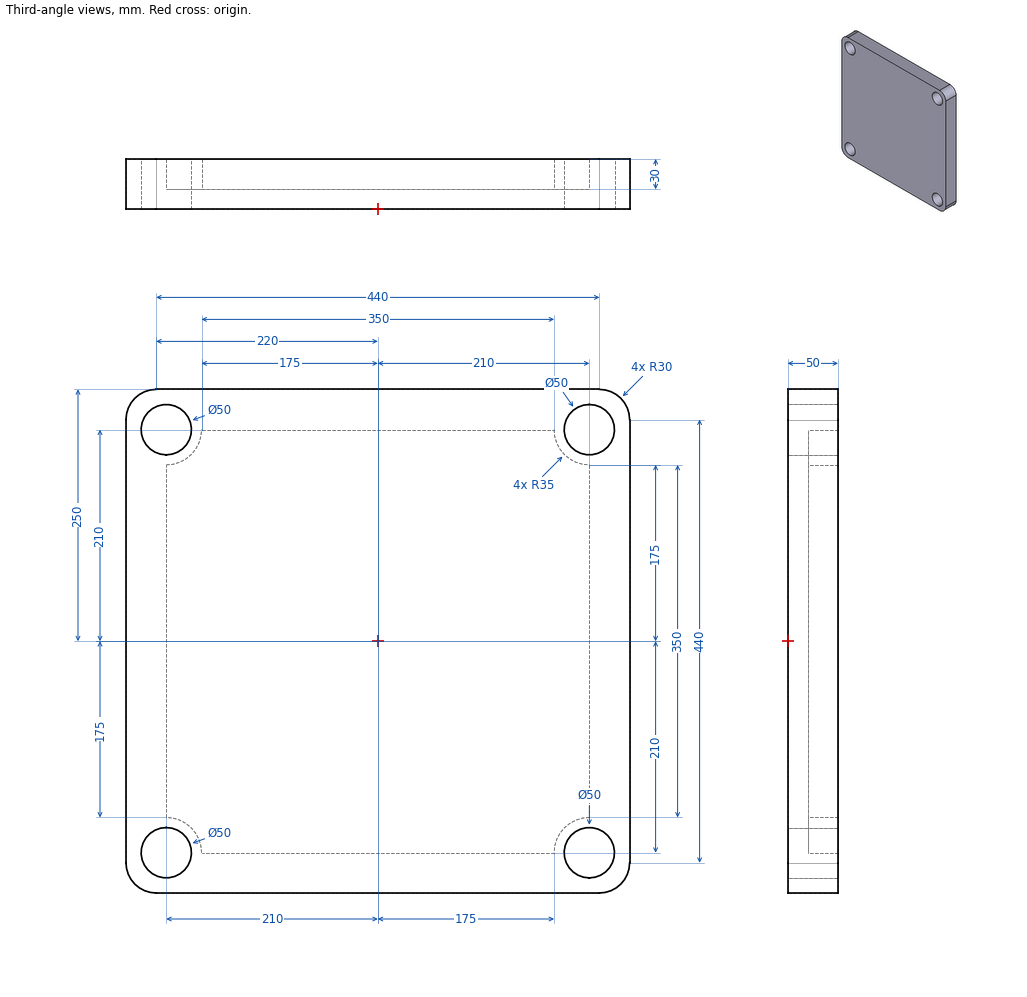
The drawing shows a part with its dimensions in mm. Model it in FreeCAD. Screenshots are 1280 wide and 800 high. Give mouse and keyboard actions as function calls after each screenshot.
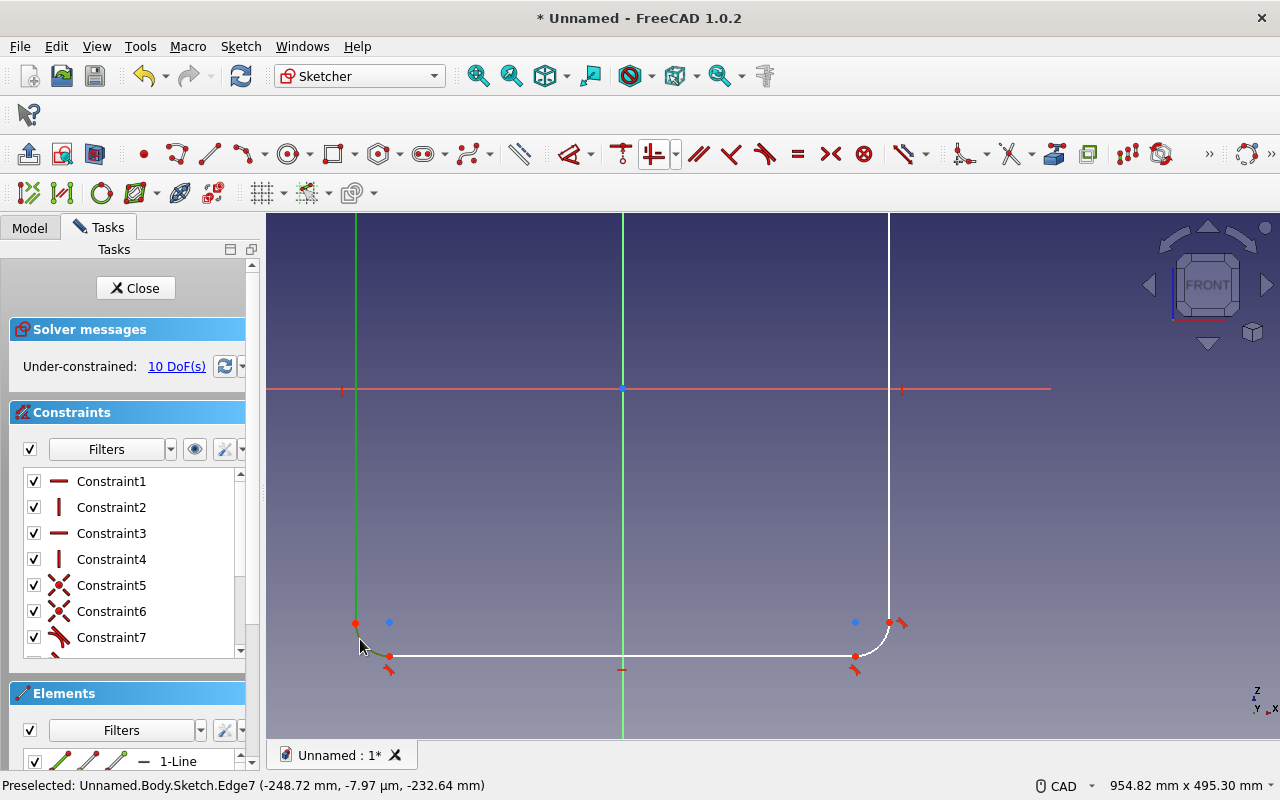
click(765, 154)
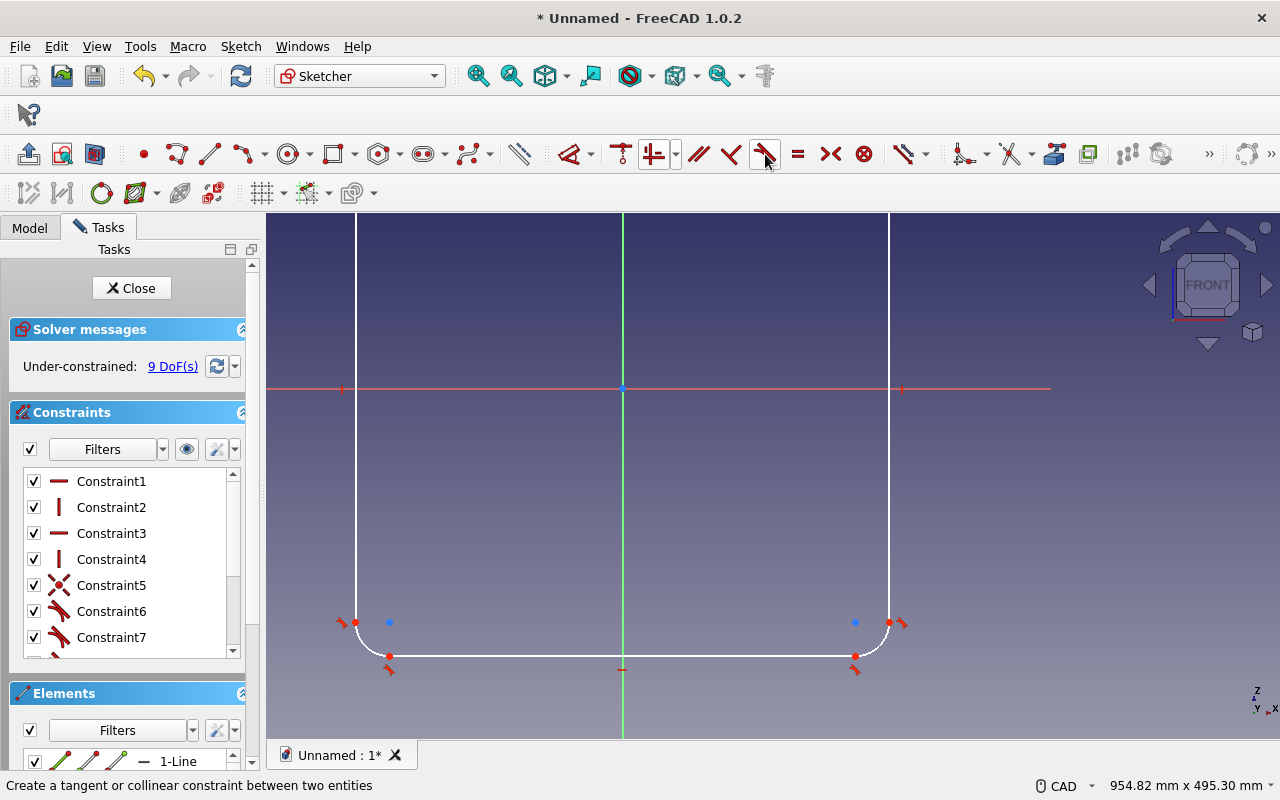
click(356, 483)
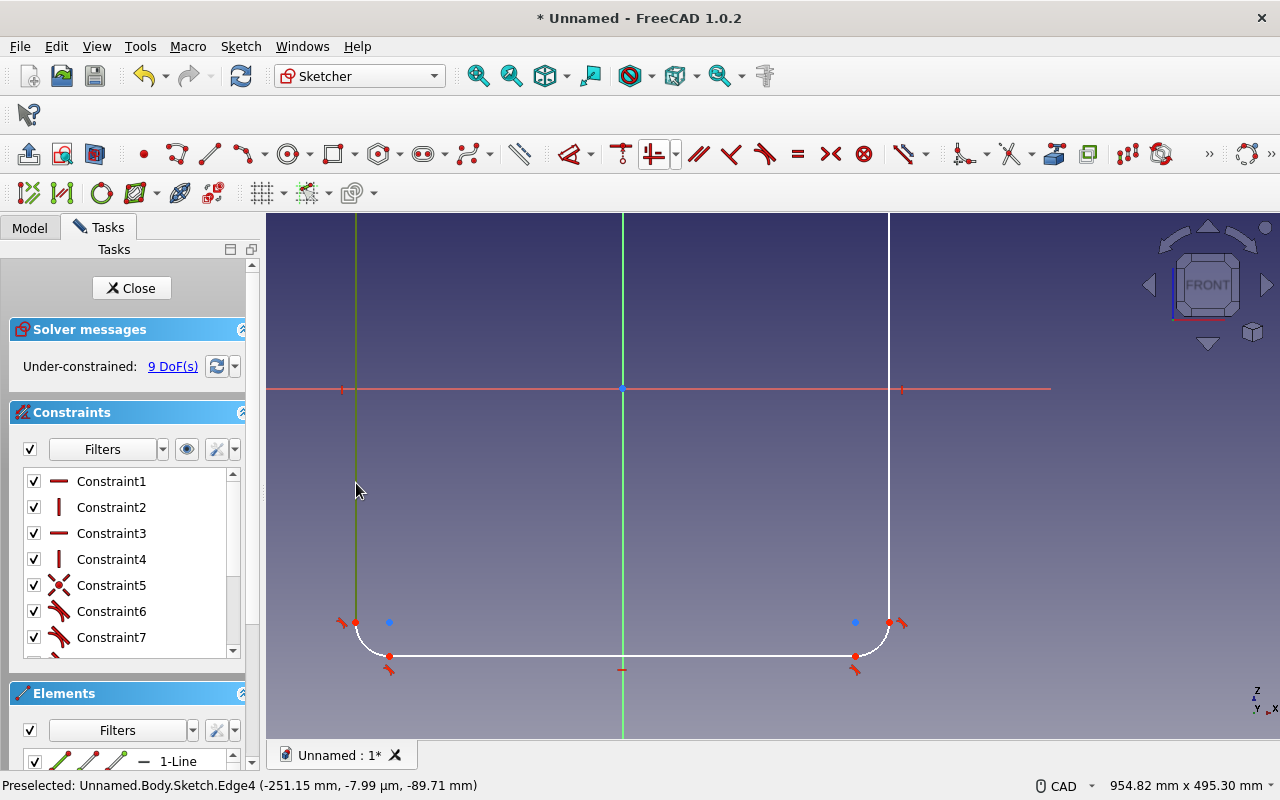
scroll(871, 653, down, 2)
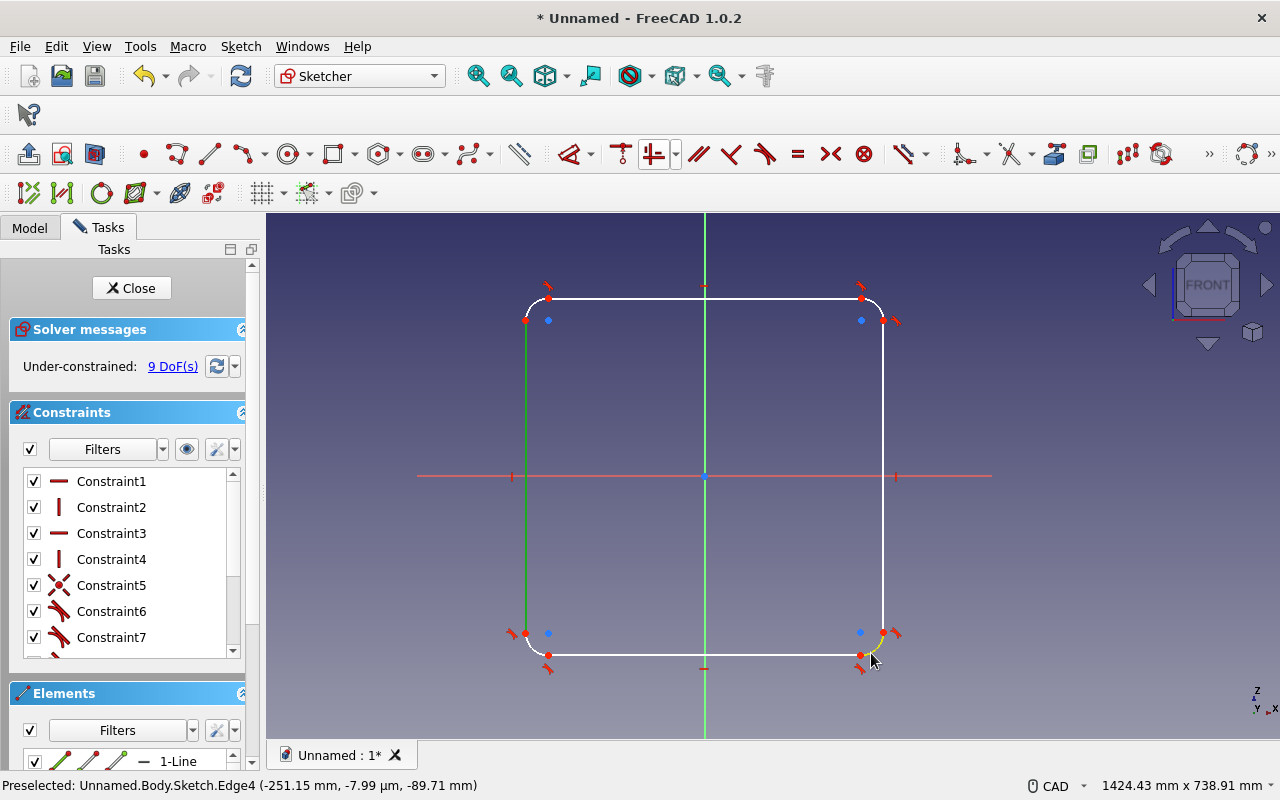
scroll(538, 301, up, 2)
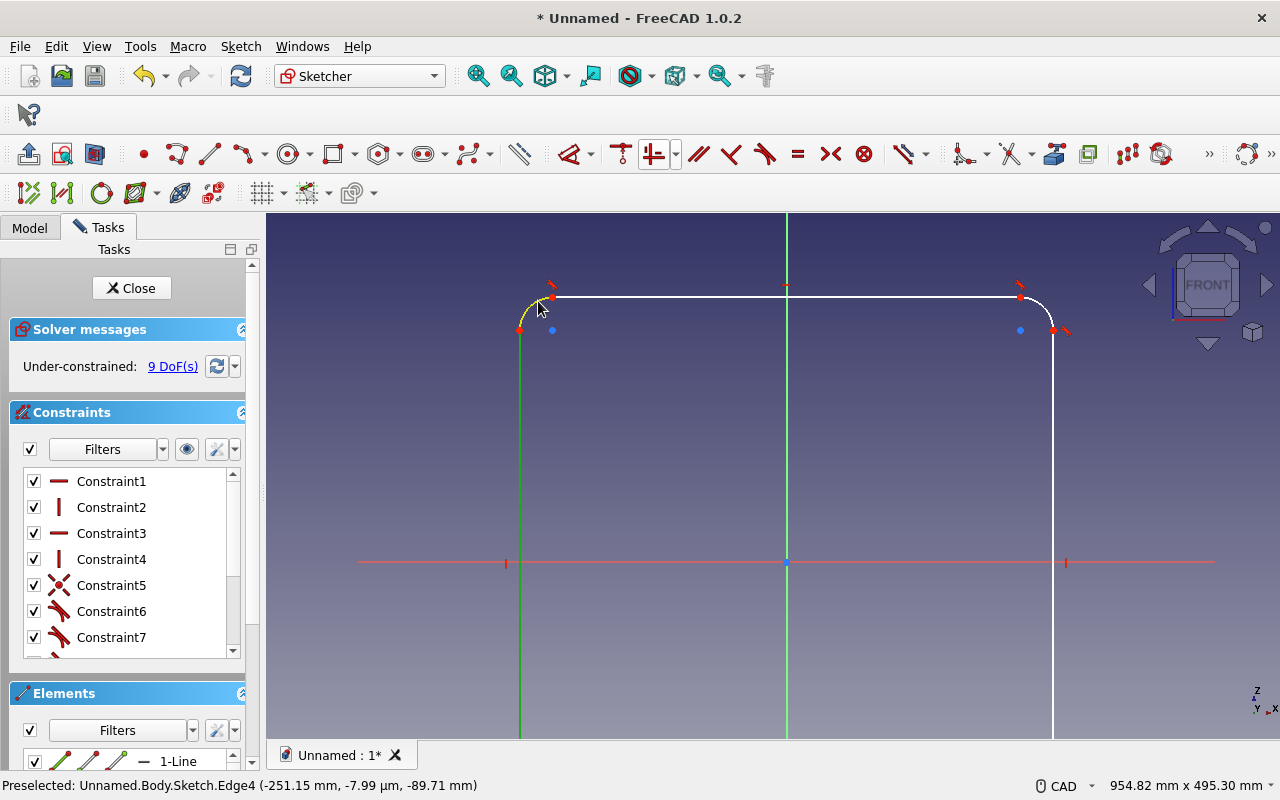
click(538, 301)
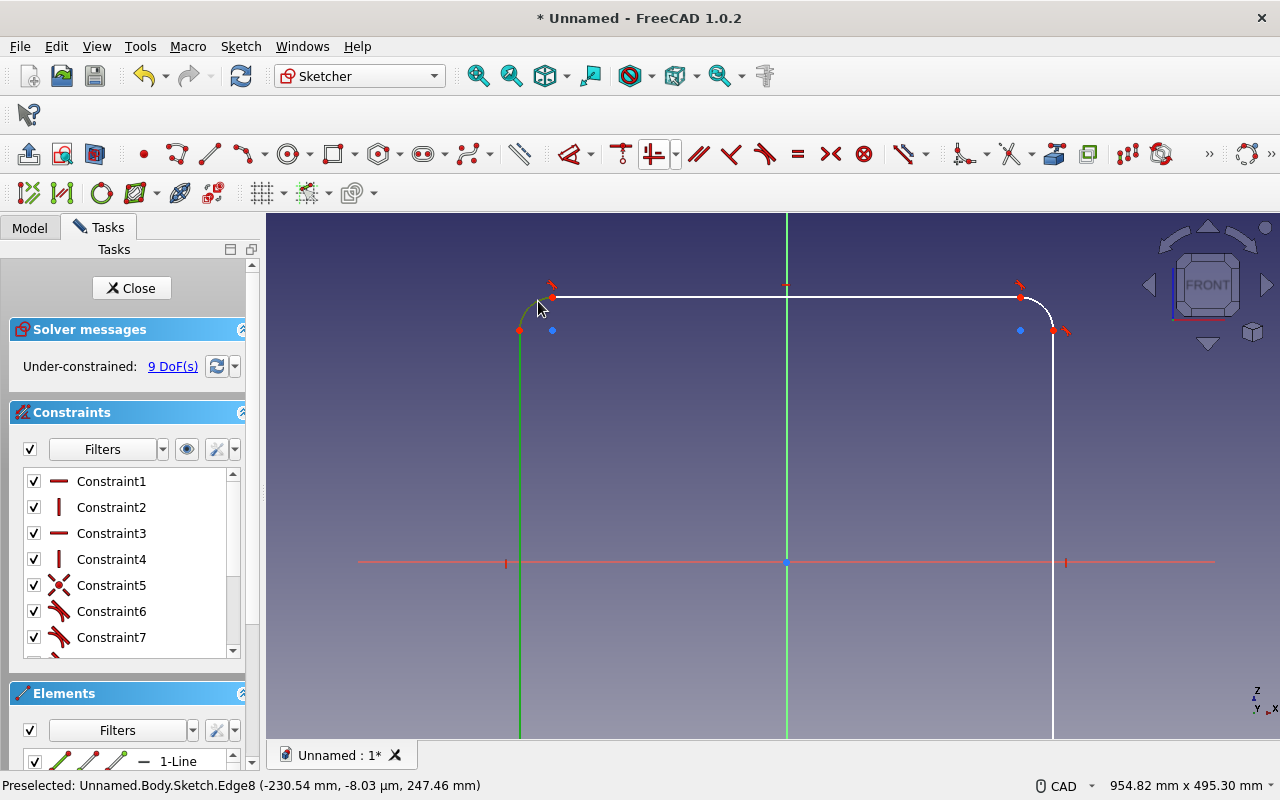
click(765, 154)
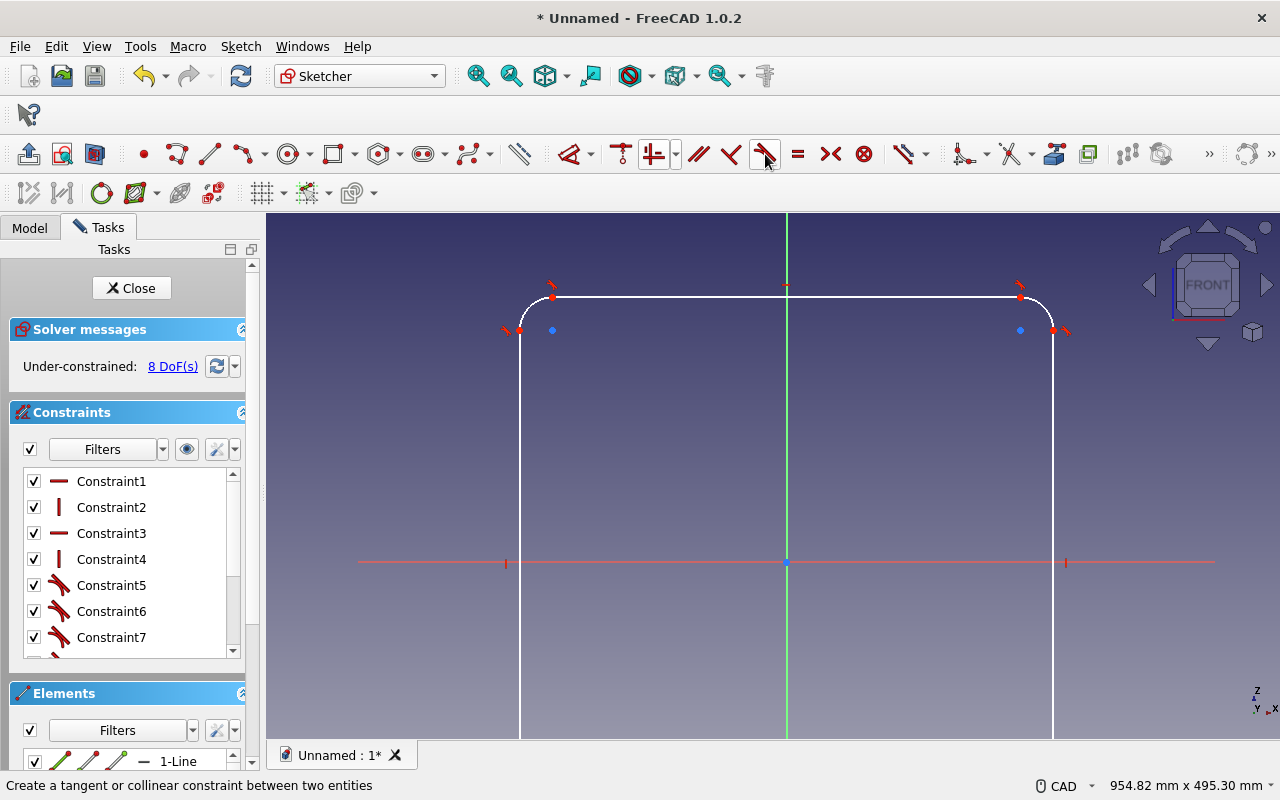
click(1050, 315)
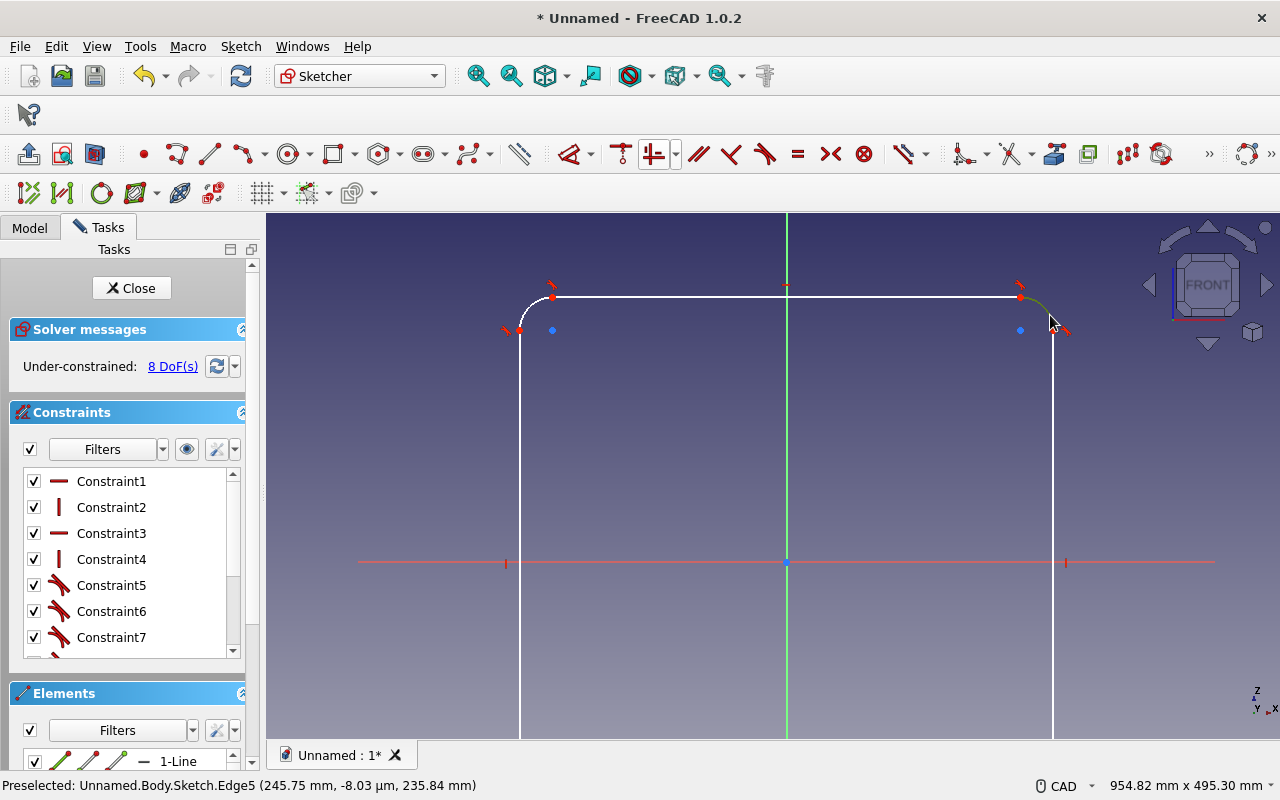
scroll(537, 301, down, 2)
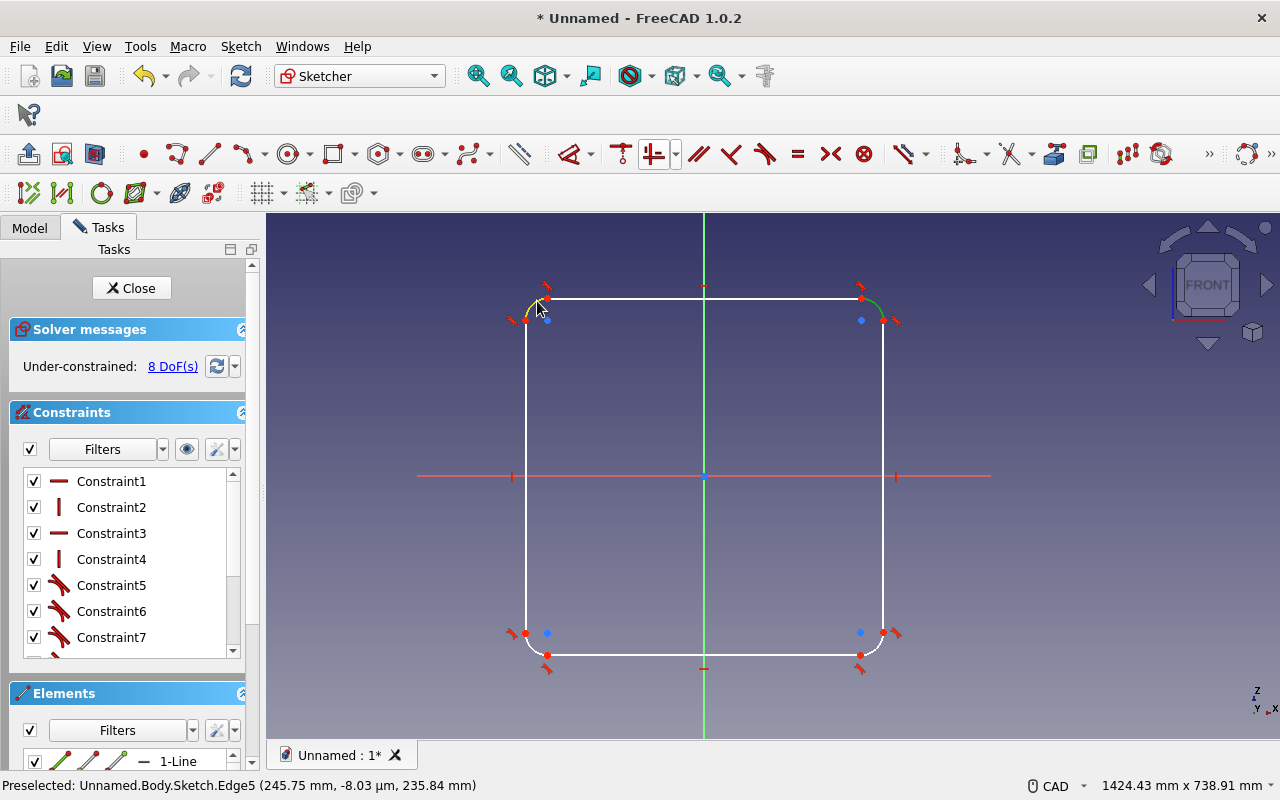
scroll(871, 653, up, 2)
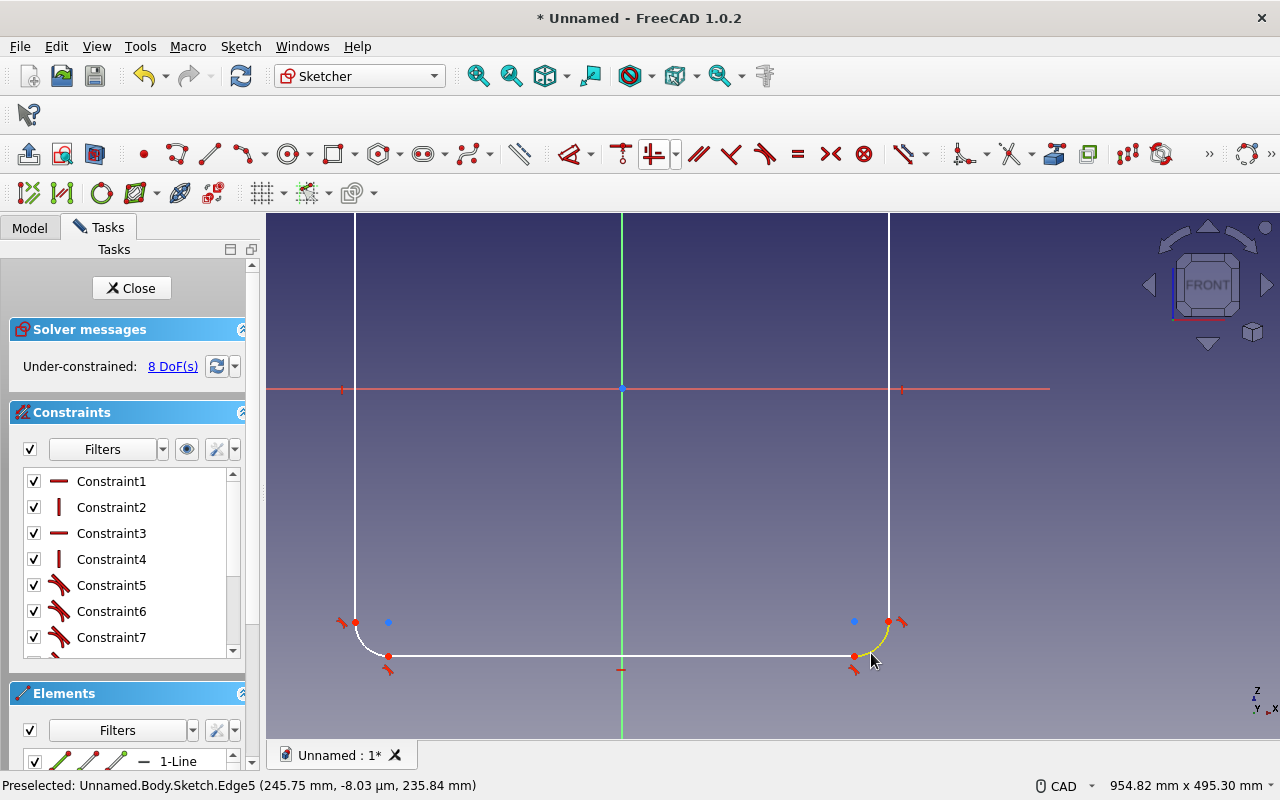
click(870, 652)